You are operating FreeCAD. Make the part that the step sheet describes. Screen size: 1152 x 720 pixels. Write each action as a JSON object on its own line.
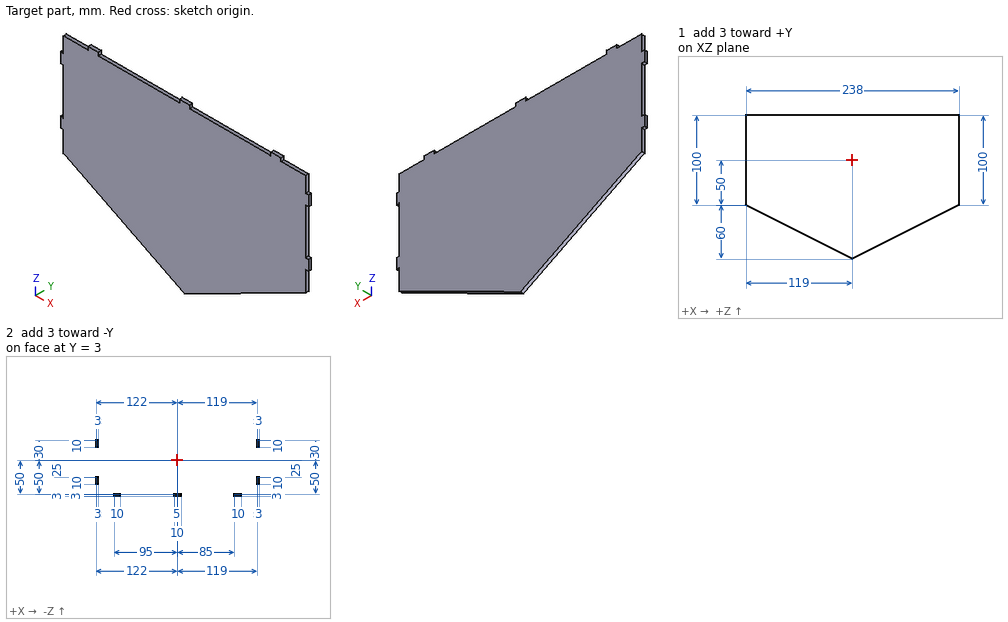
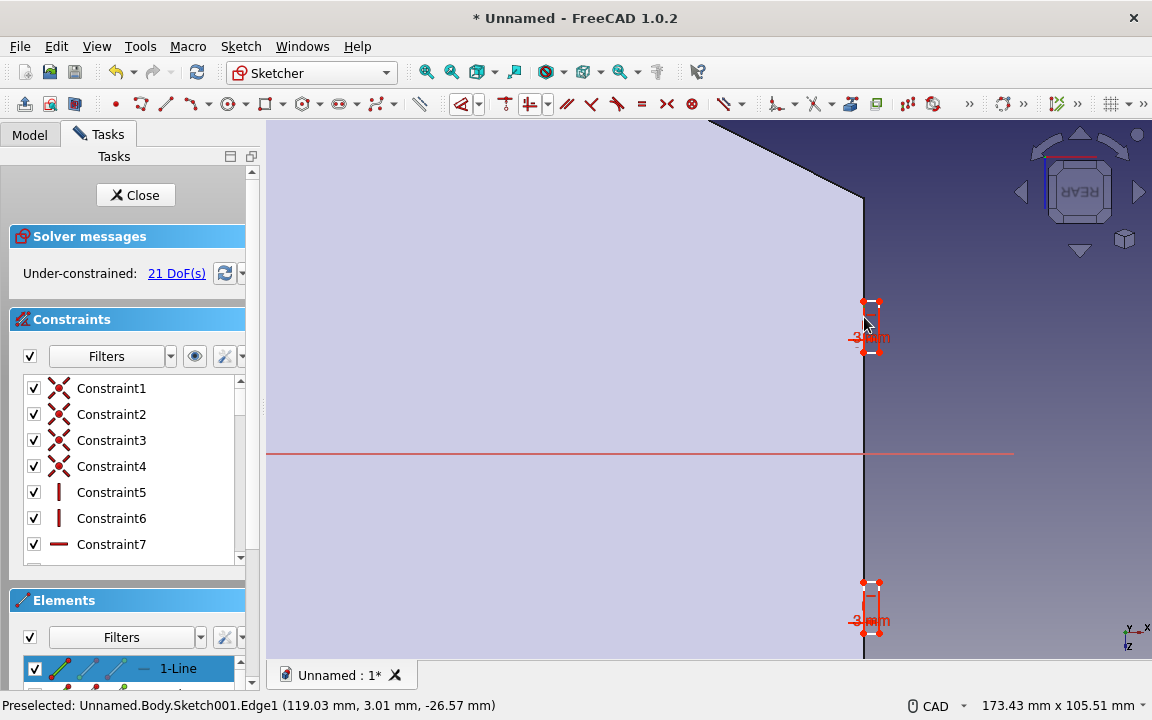
{"action": "left_click", "coordinate": [478, 104]}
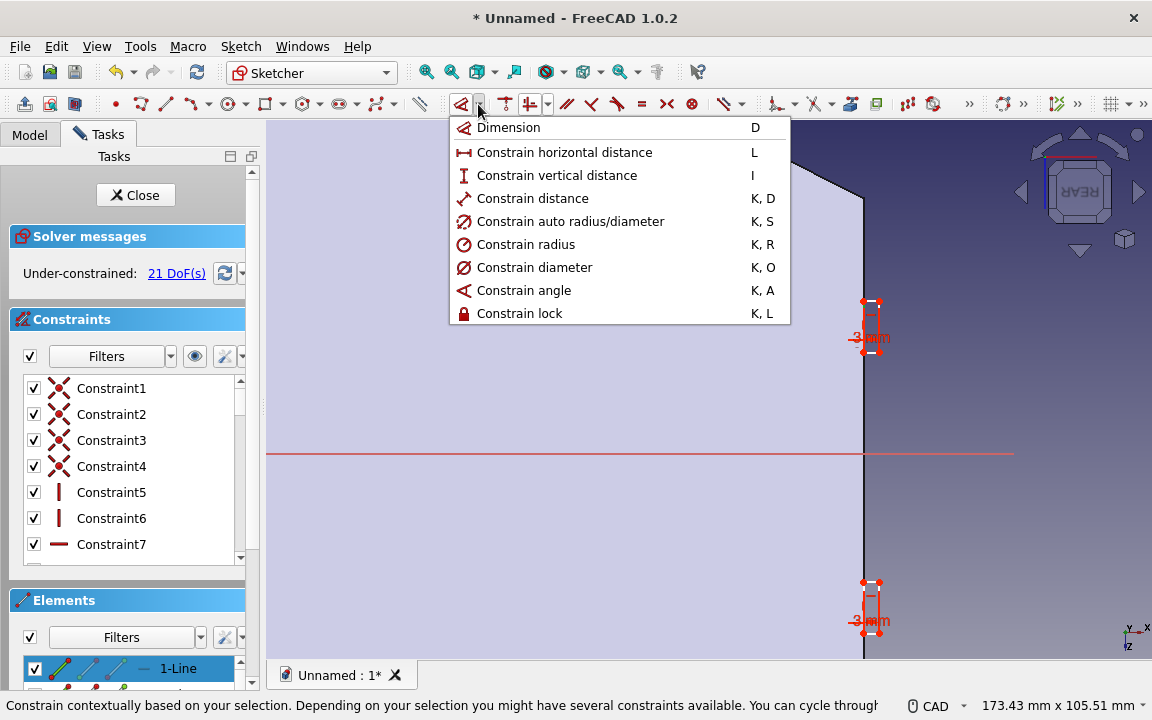
{"action": "left_click", "coordinate": [620, 176]}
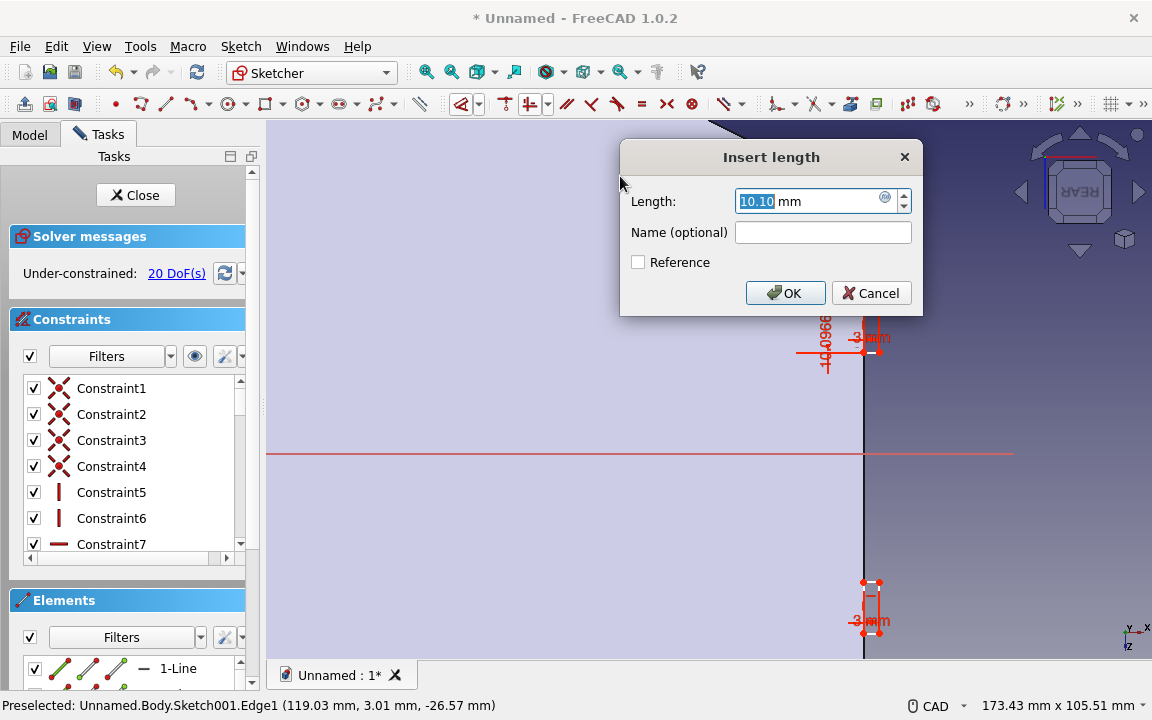
{"action": "type", "text": "10"}
{"action": "key", "text": "Return"}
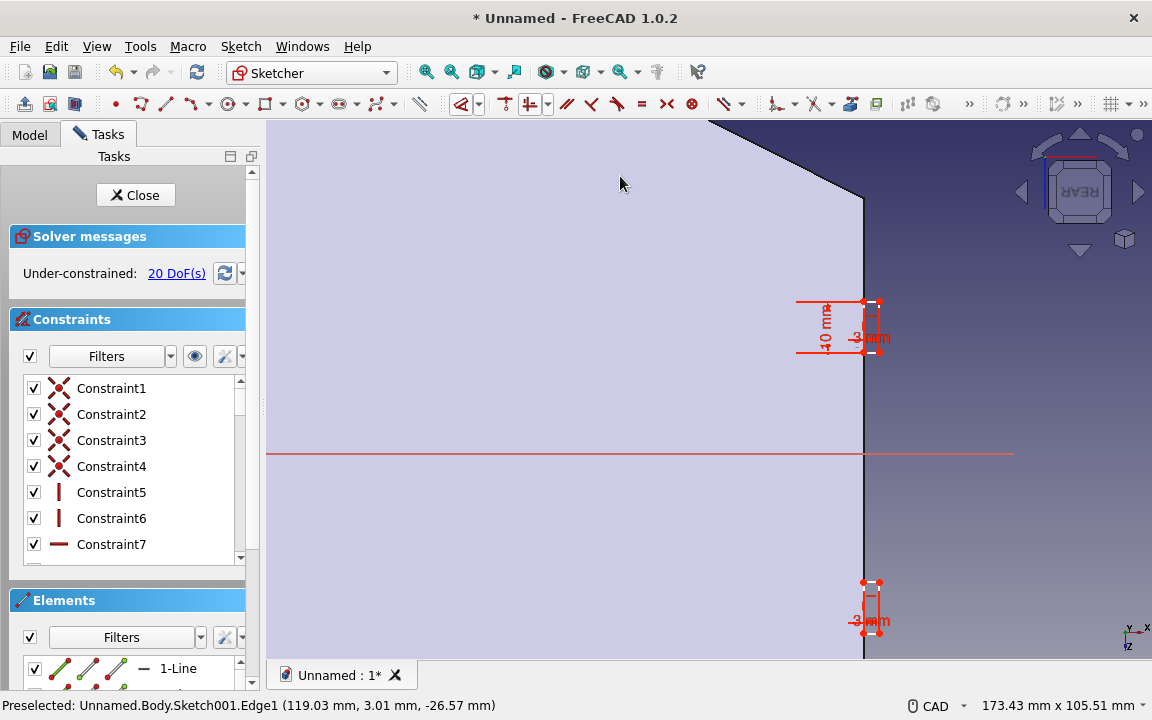
{"action": "left_click", "coordinate": [864, 598]}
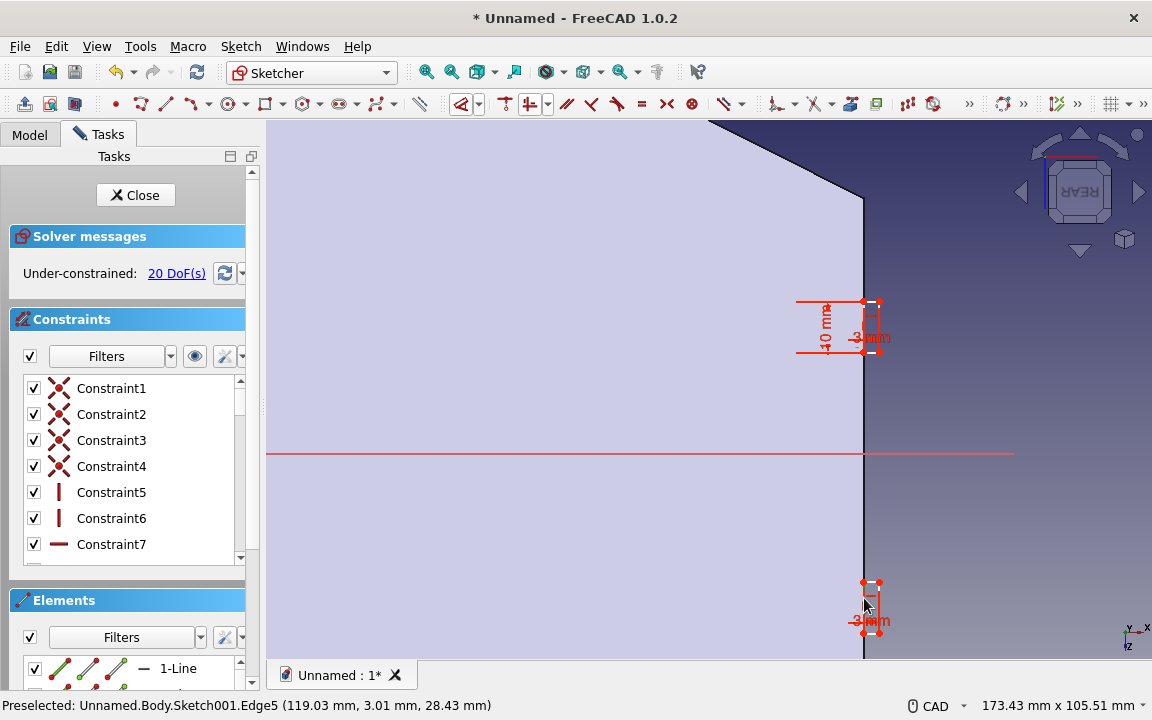
{"action": "key", "text": "i"}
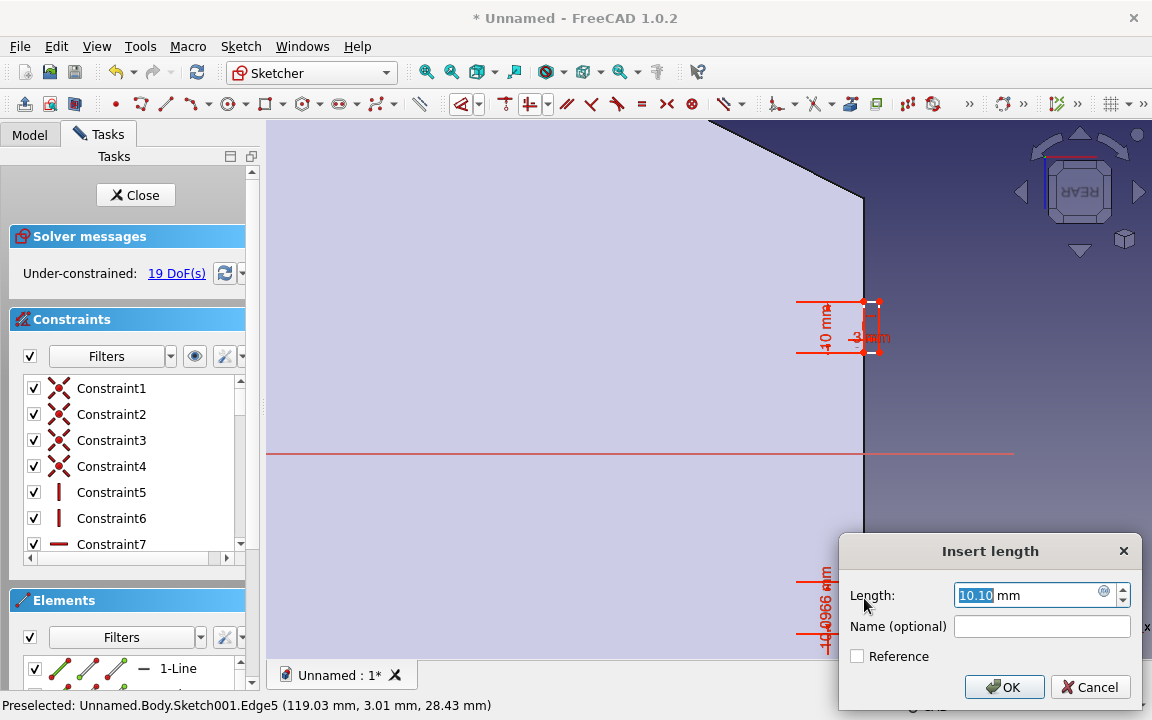
{"action": "type", "text": "10"}
{"action": "key", "text": "Return"}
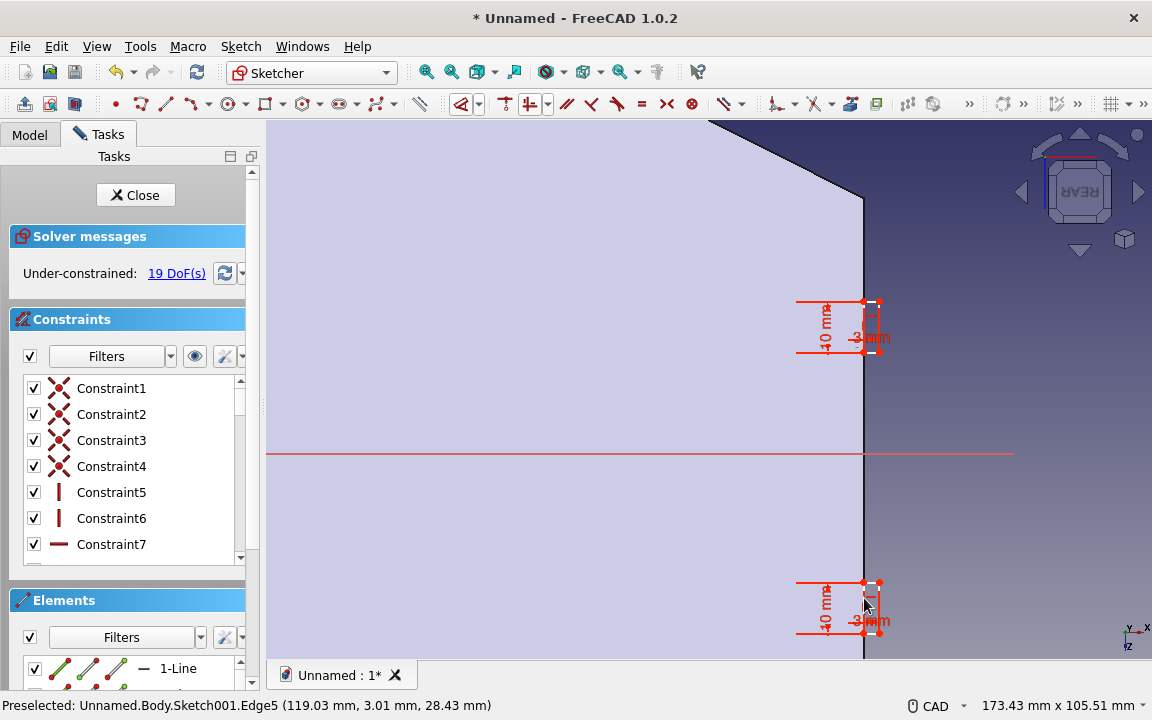
{"action": "scroll", "coordinate": [864, 318], "scroll_direction": "down", "scroll_amount": 5}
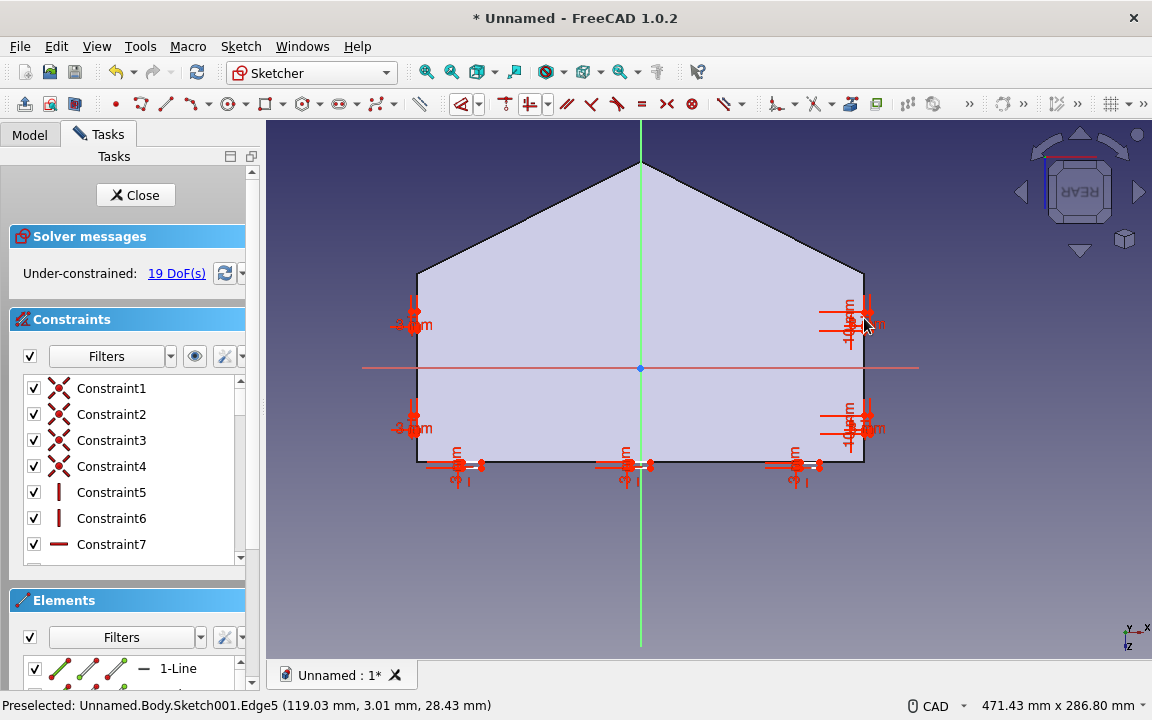
{"action": "scroll", "coordinate": [411, 421], "scroll_direction": "up", "scroll_amount": 5}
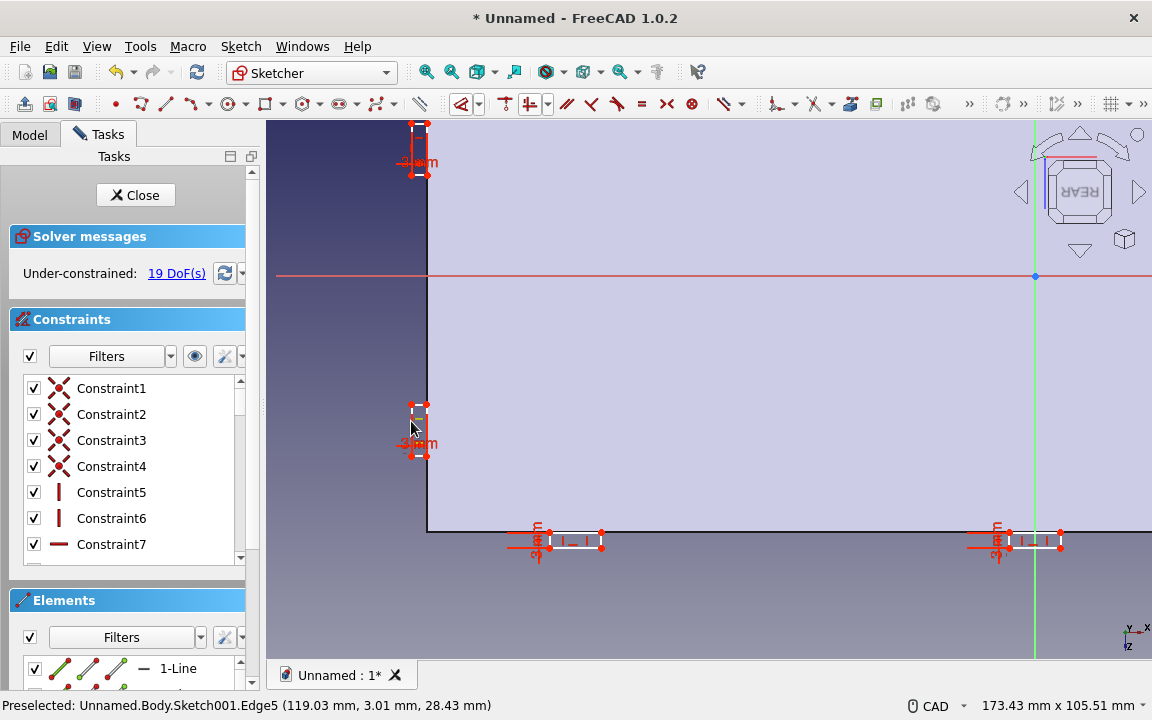
{"action": "left_click", "coordinate": [412, 420]}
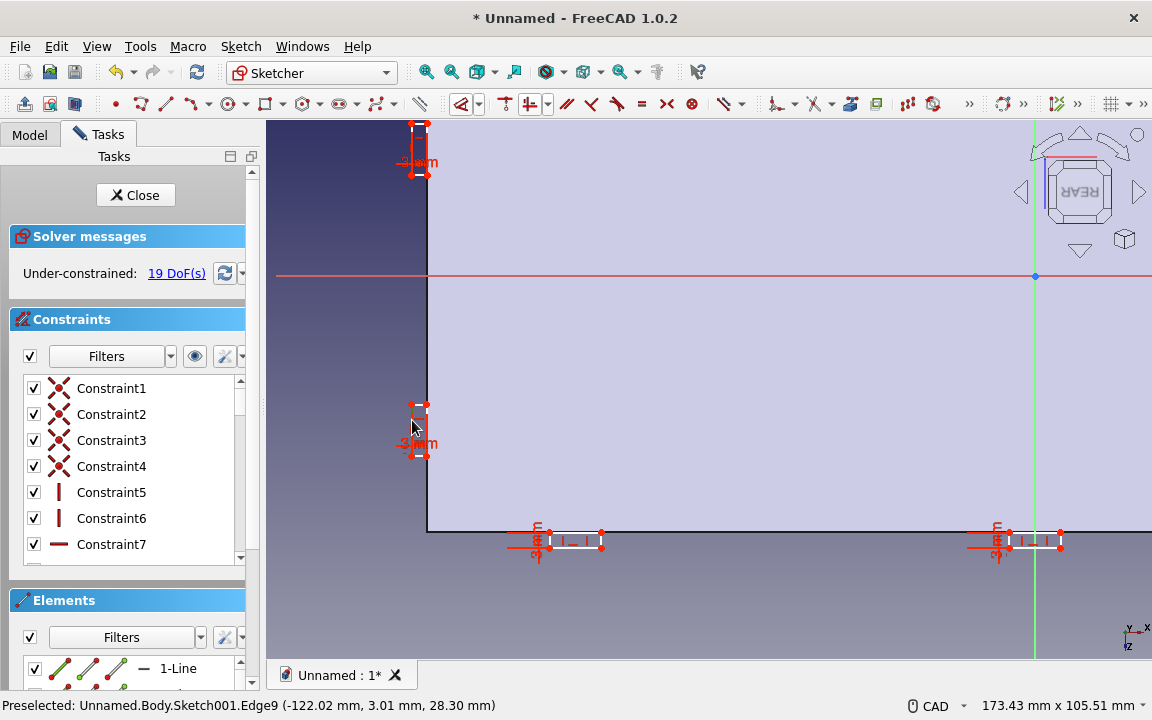
{"action": "key", "text": "i"}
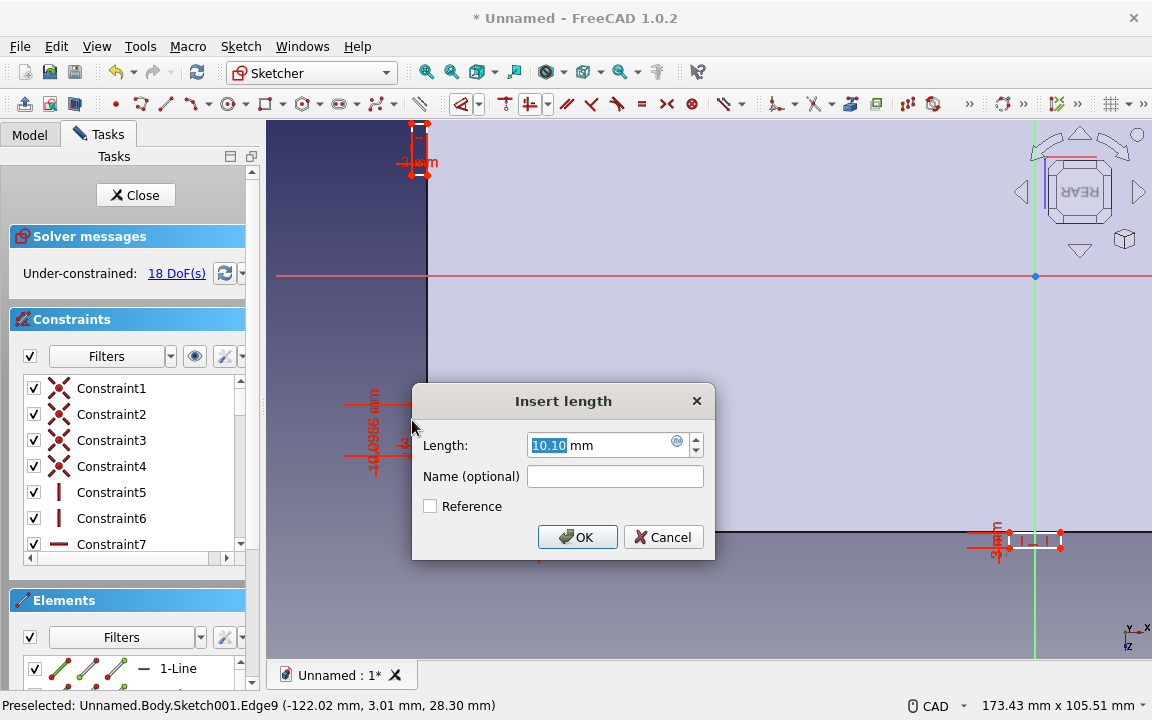
{"action": "type", "text": "10"}
{"action": "key", "text": "Return"}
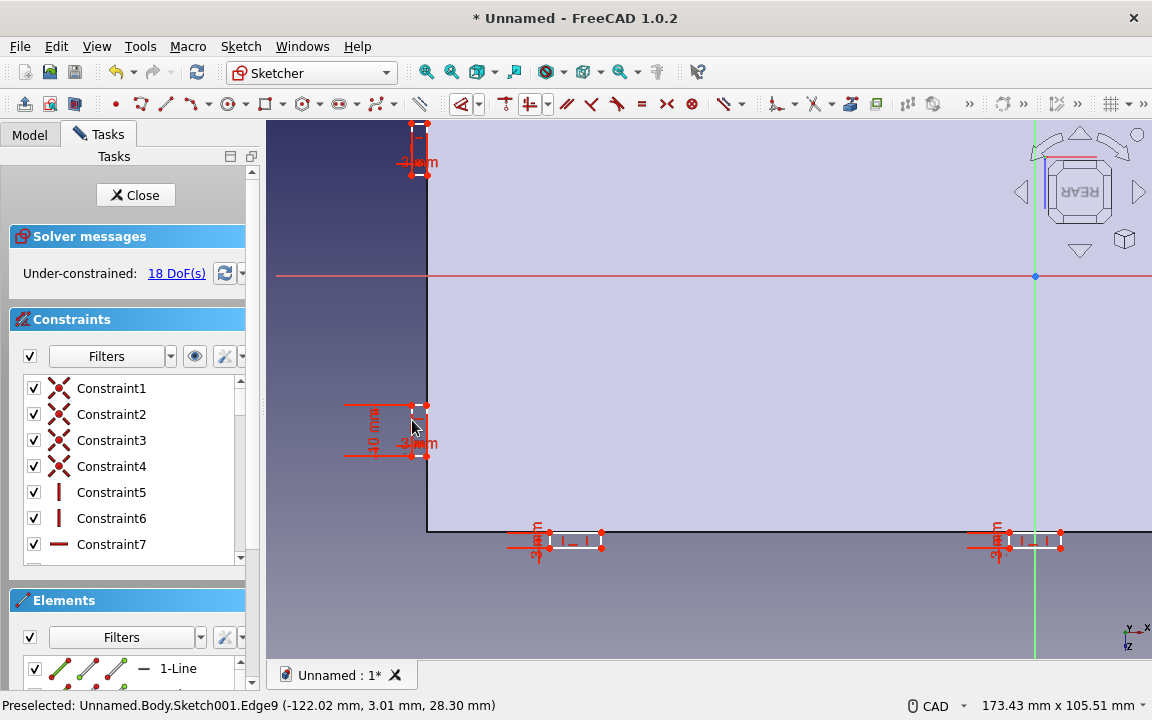
{"action": "scroll", "coordinate": [412, 160], "scroll_direction": "up", "scroll_amount": 4}